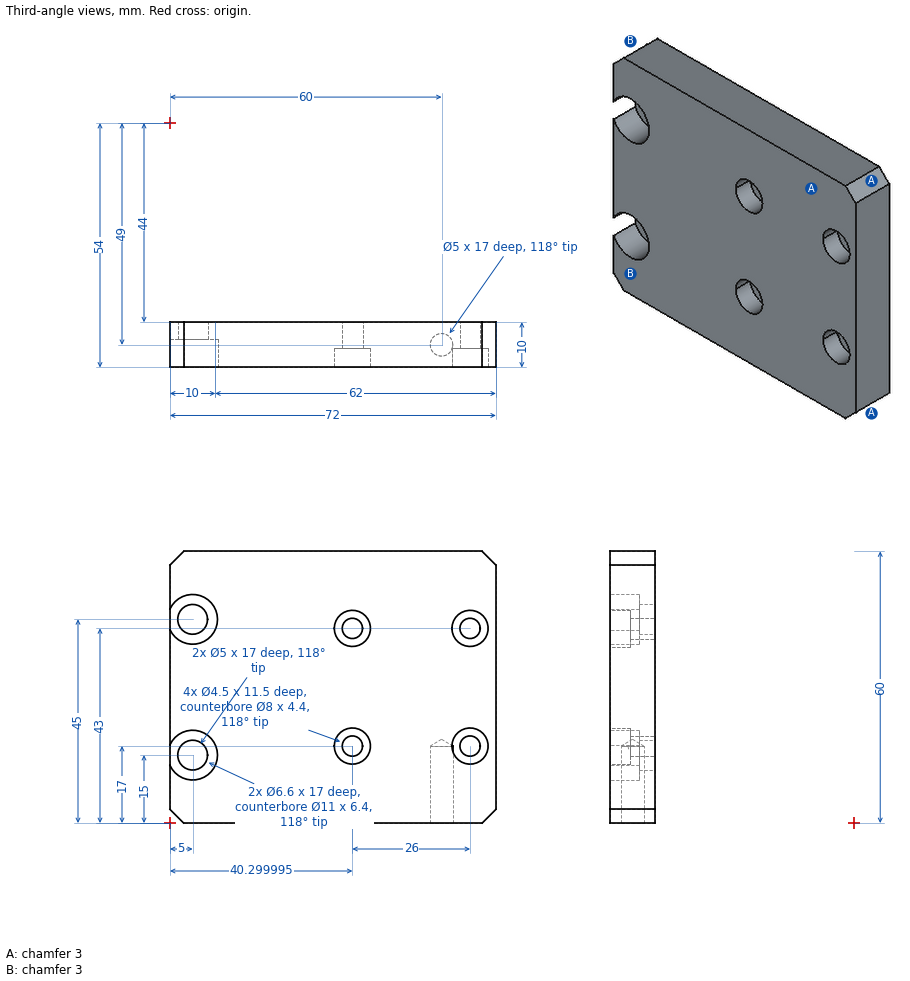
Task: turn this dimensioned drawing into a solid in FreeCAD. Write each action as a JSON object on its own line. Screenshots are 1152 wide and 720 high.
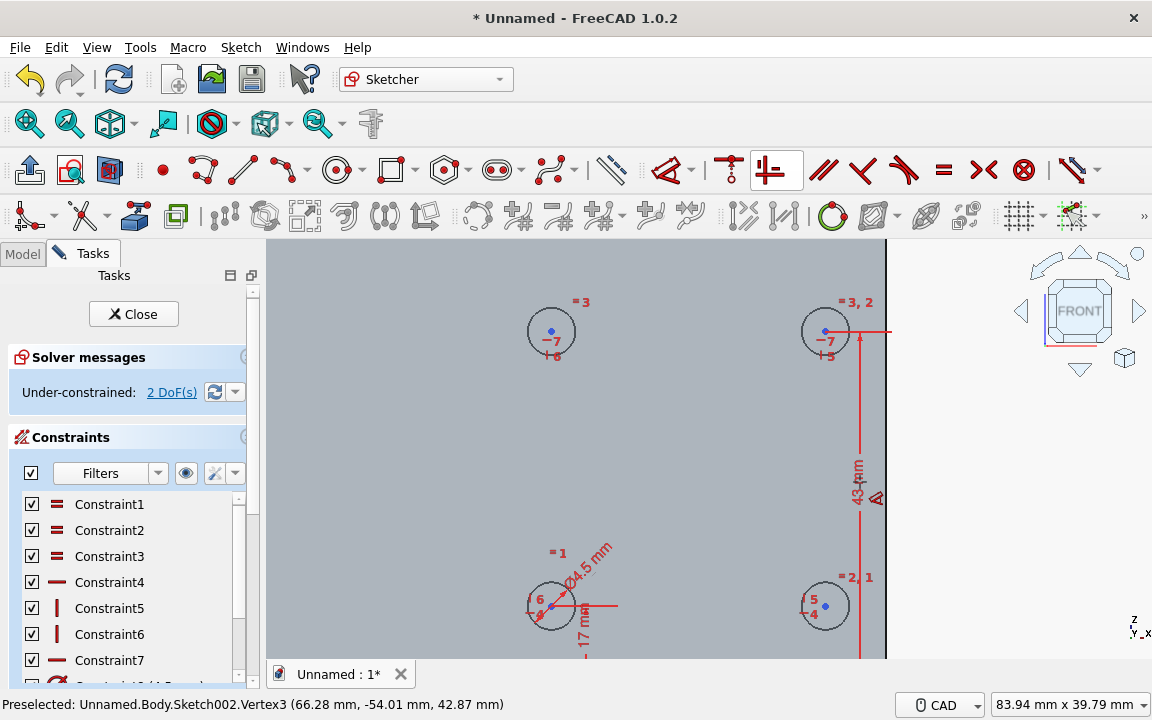
{"action": "left_click", "coordinate": [552, 606]}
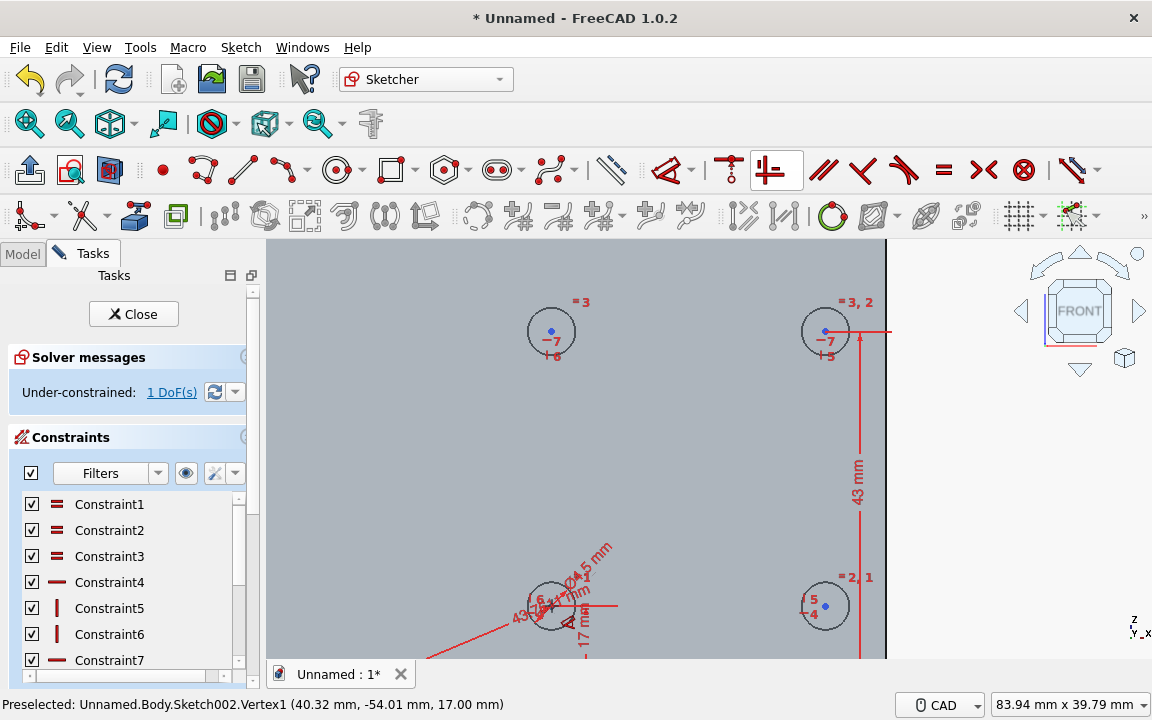
{"action": "left_click", "coordinate": [826, 606]}
{"action": "left_click", "coordinate": [689, 572]}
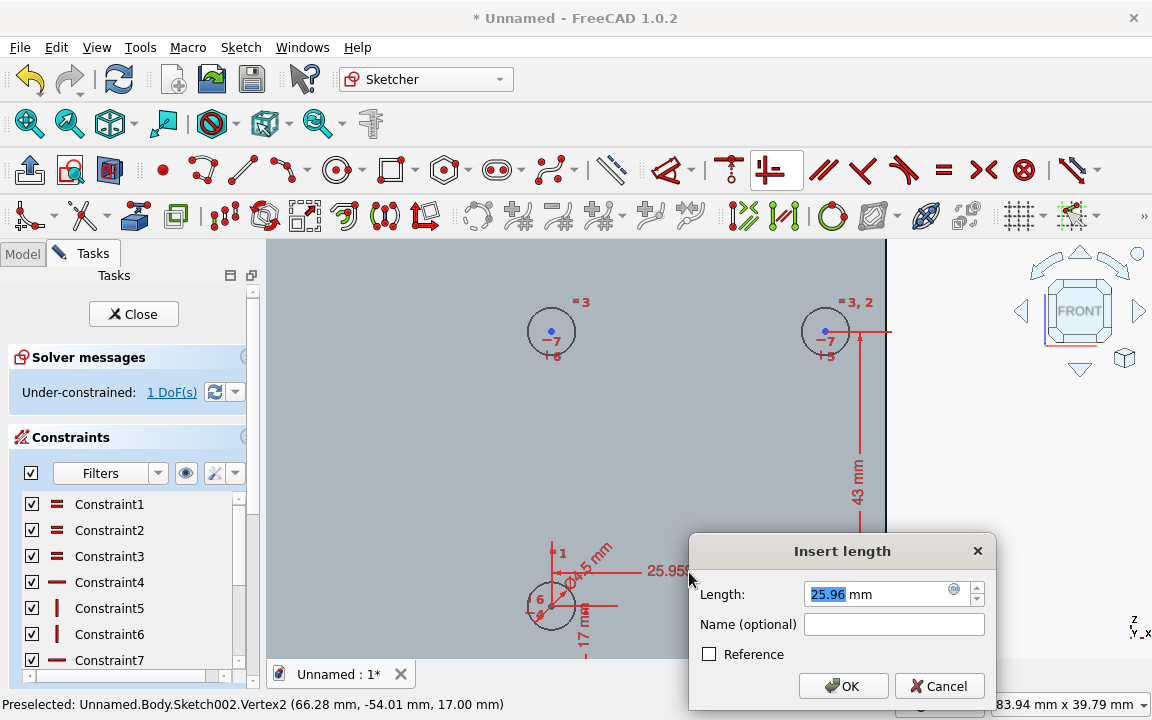
{"action": "type", "text": "26"}
{"action": "key", "text": "Return"}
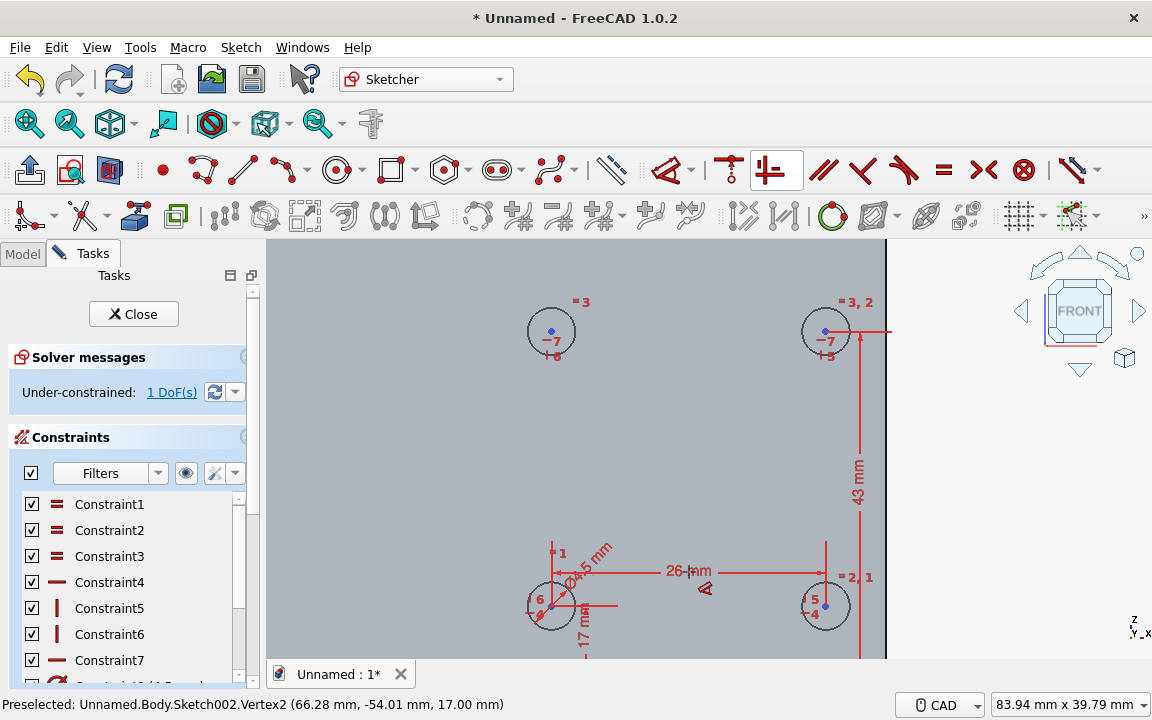
{"action": "left_click", "coordinate": [552, 606]}
{"action": "left_click", "coordinate": [423, 572]}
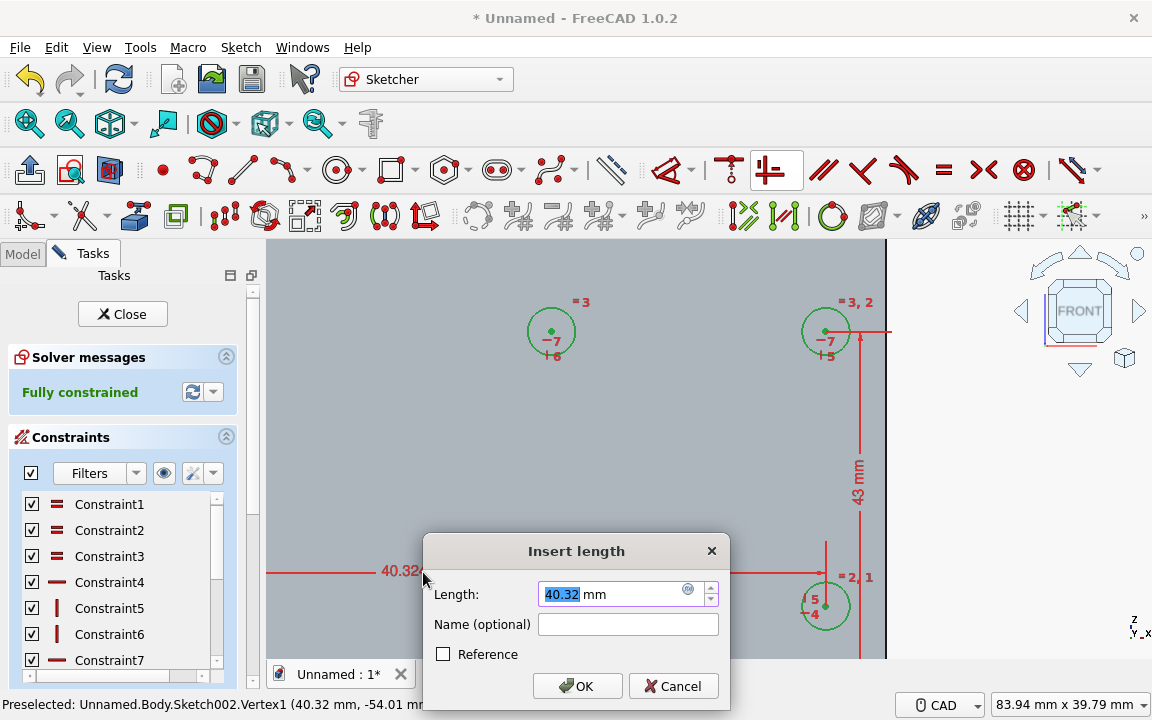
{"action": "type", "text": "40.299995"}
{"action": "key", "text": "Return"}
{"action": "key", "text": "Escape"}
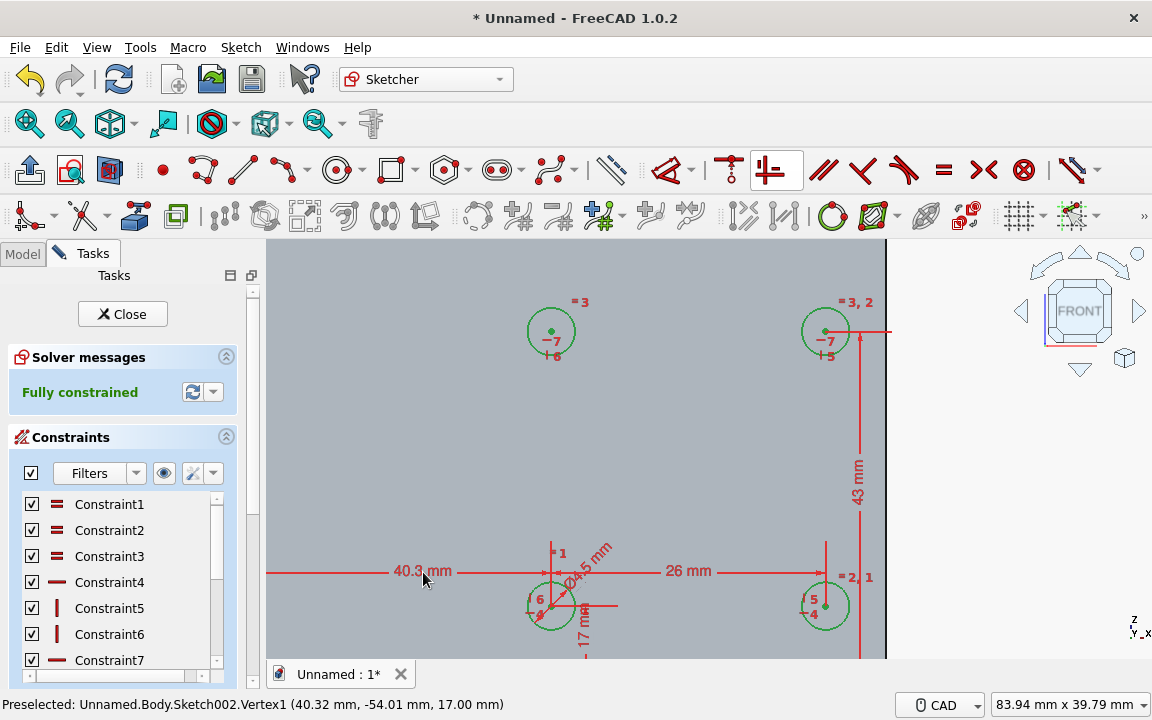
{"action": "left_click", "coordinate": [123, 314]}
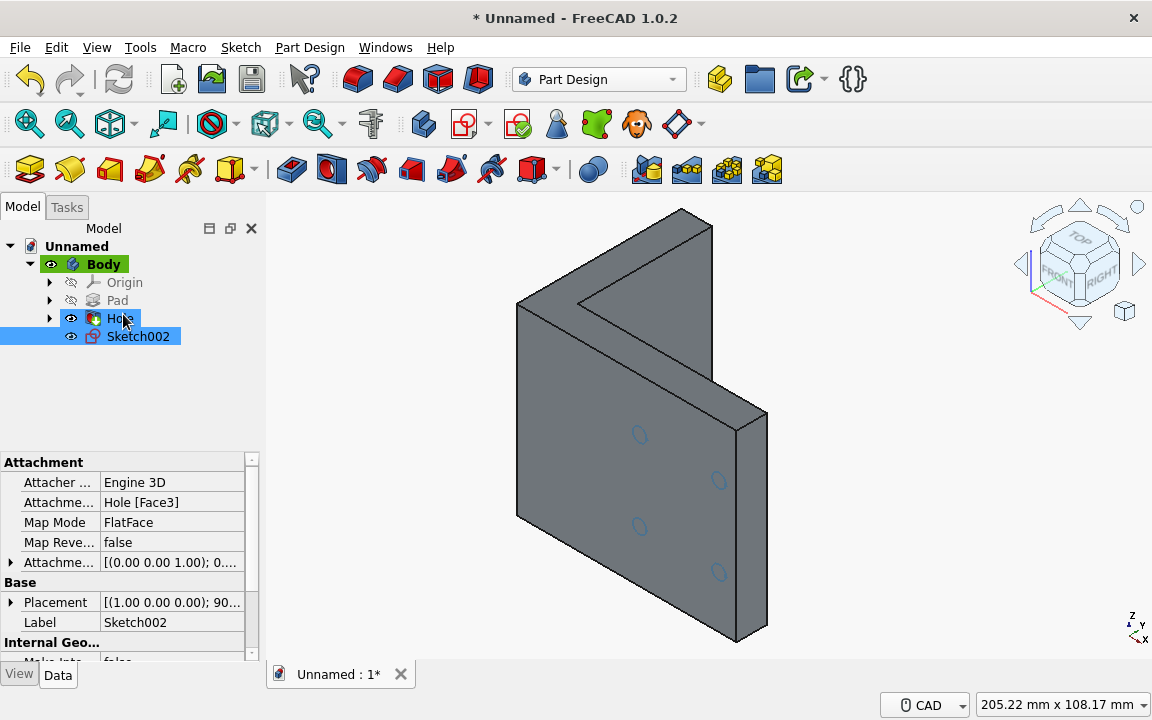
{"action": "left_click", "coordinate": [332, 170]}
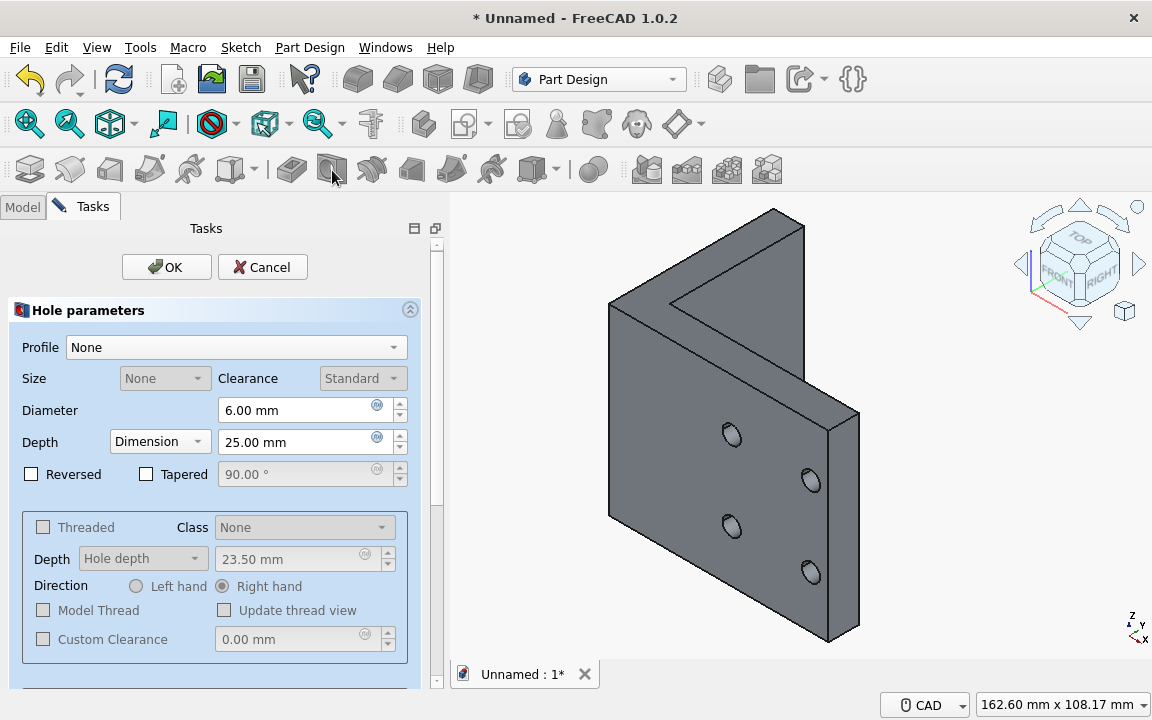
{"action": "triple_click", "coordinate": [305, 410]}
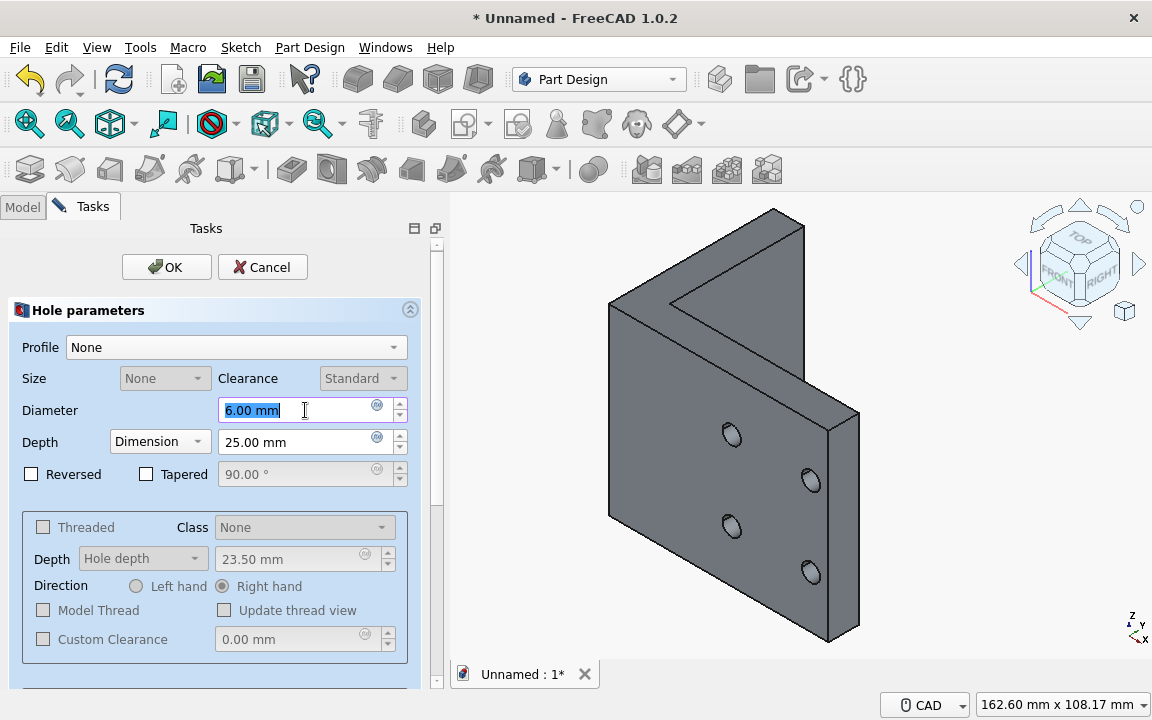
{"action": "type", "text": "4.5"}
{"action": "key", "text": "Tab"}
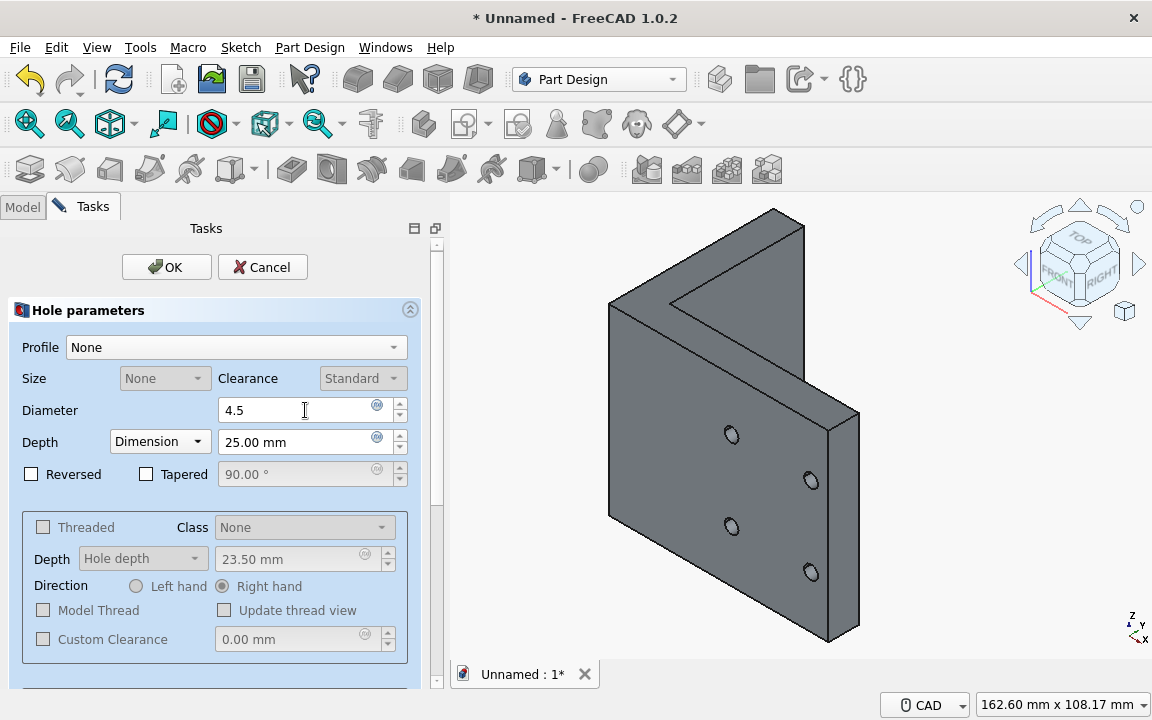
{"action": "triple_click", "coordinate": [305, 442]}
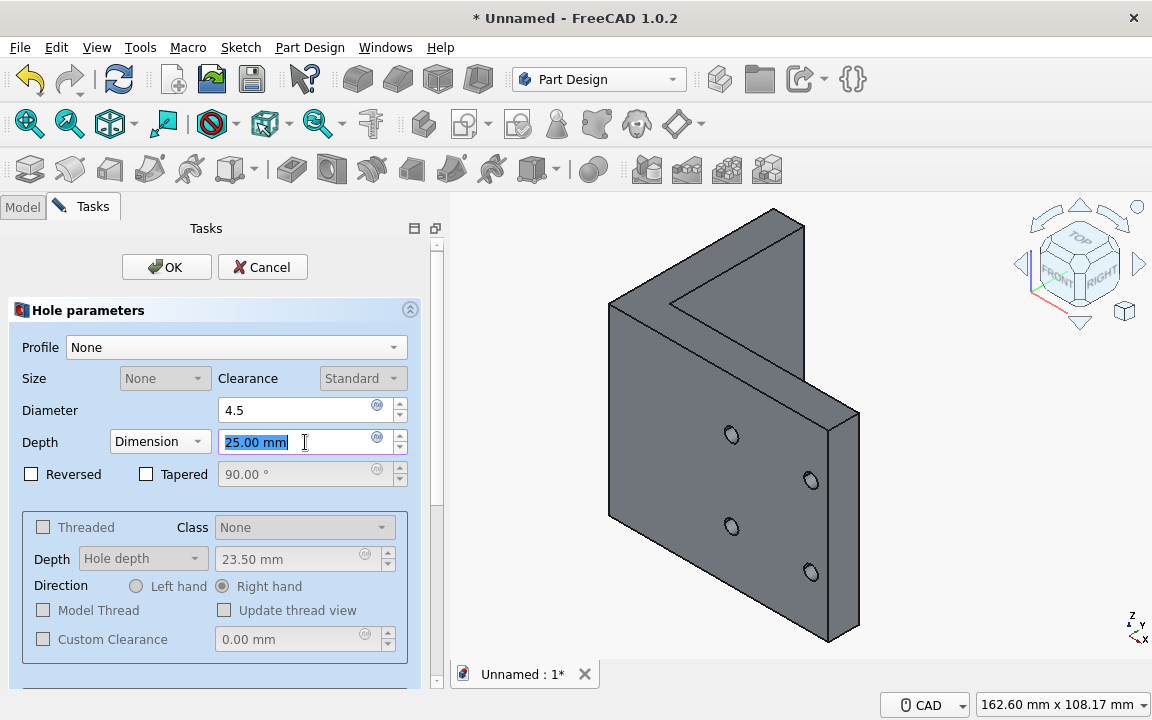
{"action": "type", "text": "11.5"}
{"action": "key", "text": "Tab"}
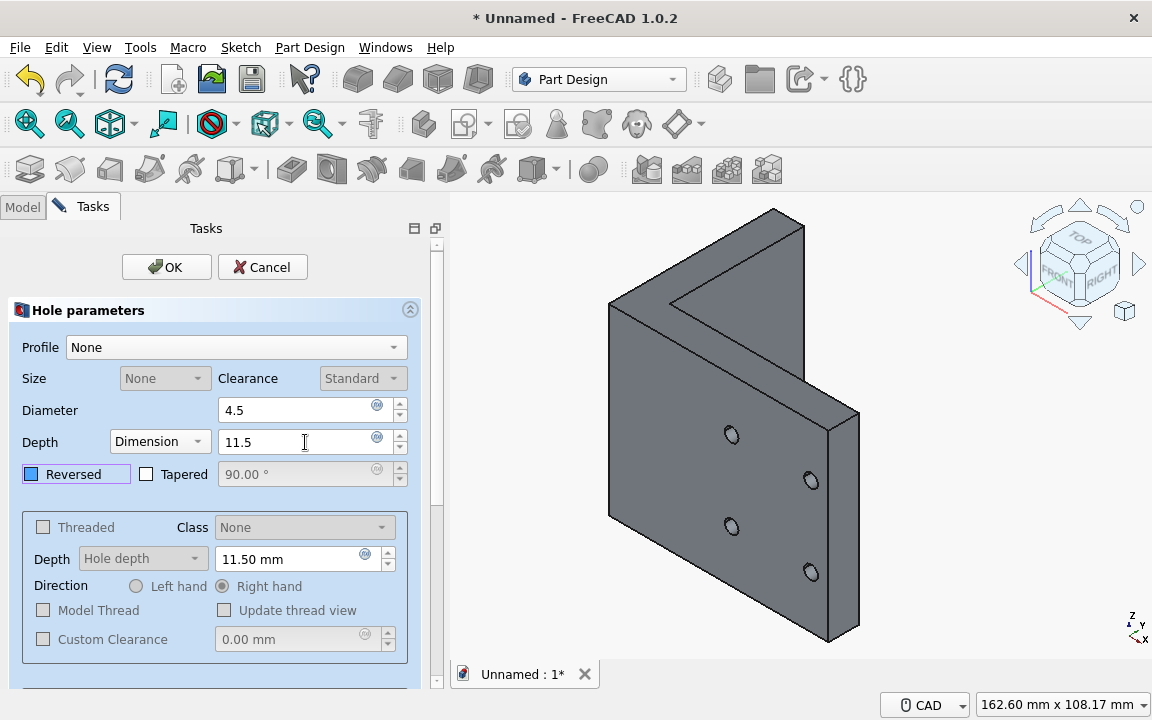
{"action": "scroll", "coordinate": [437, 463], "scroll_direction": "down", "scroll_amount": 2}